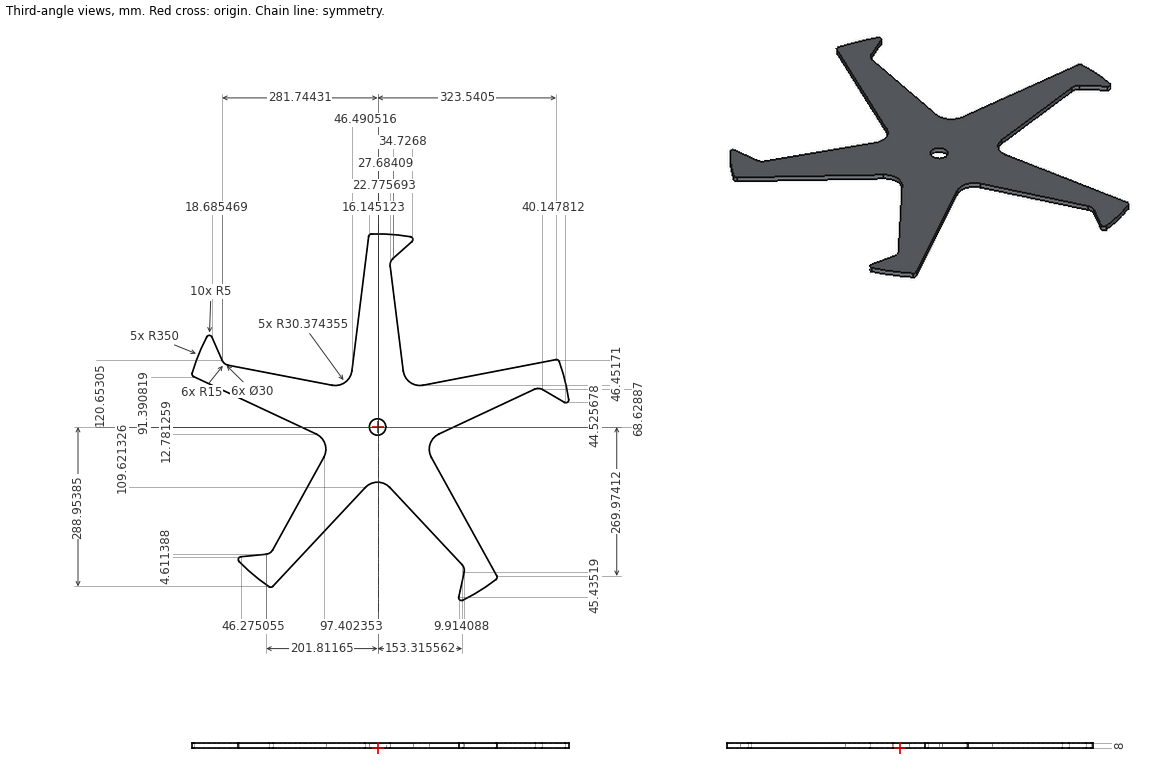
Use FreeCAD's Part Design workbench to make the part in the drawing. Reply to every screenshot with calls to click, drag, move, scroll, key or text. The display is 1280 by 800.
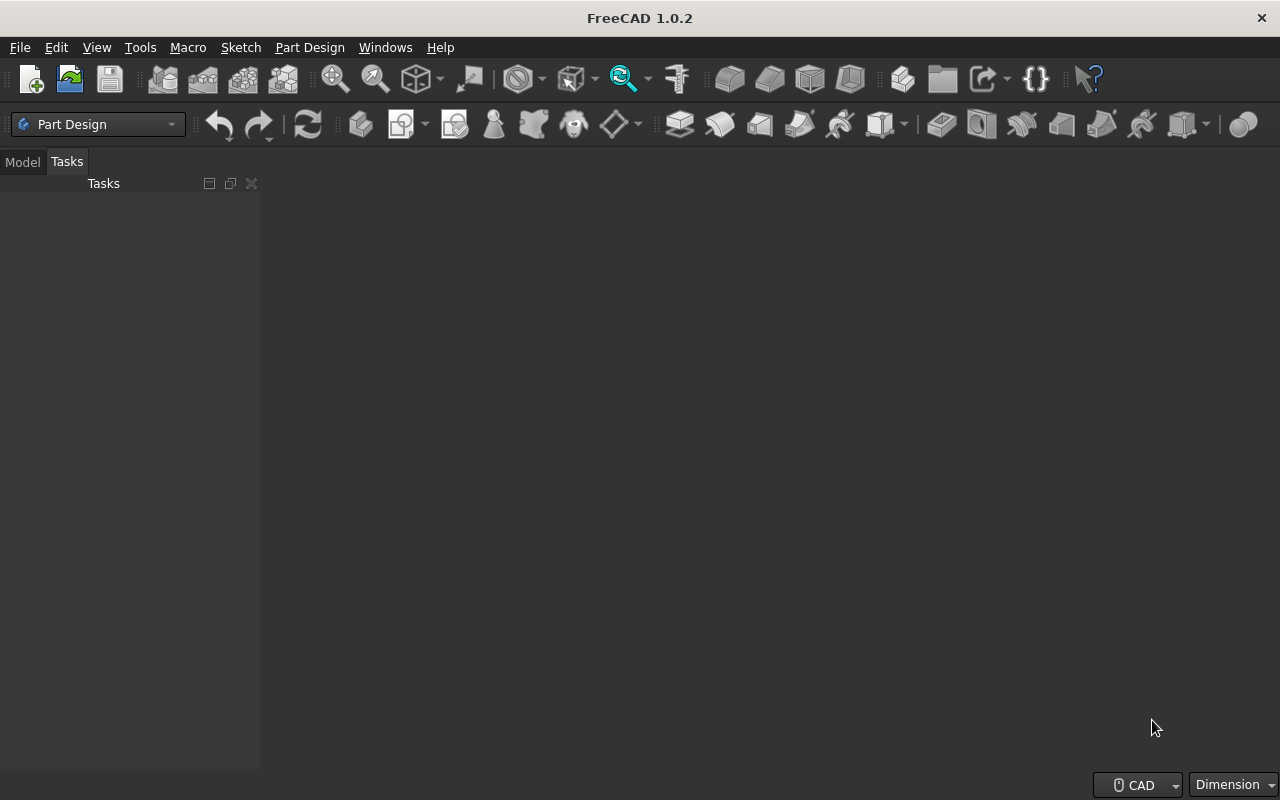
click(30, 80)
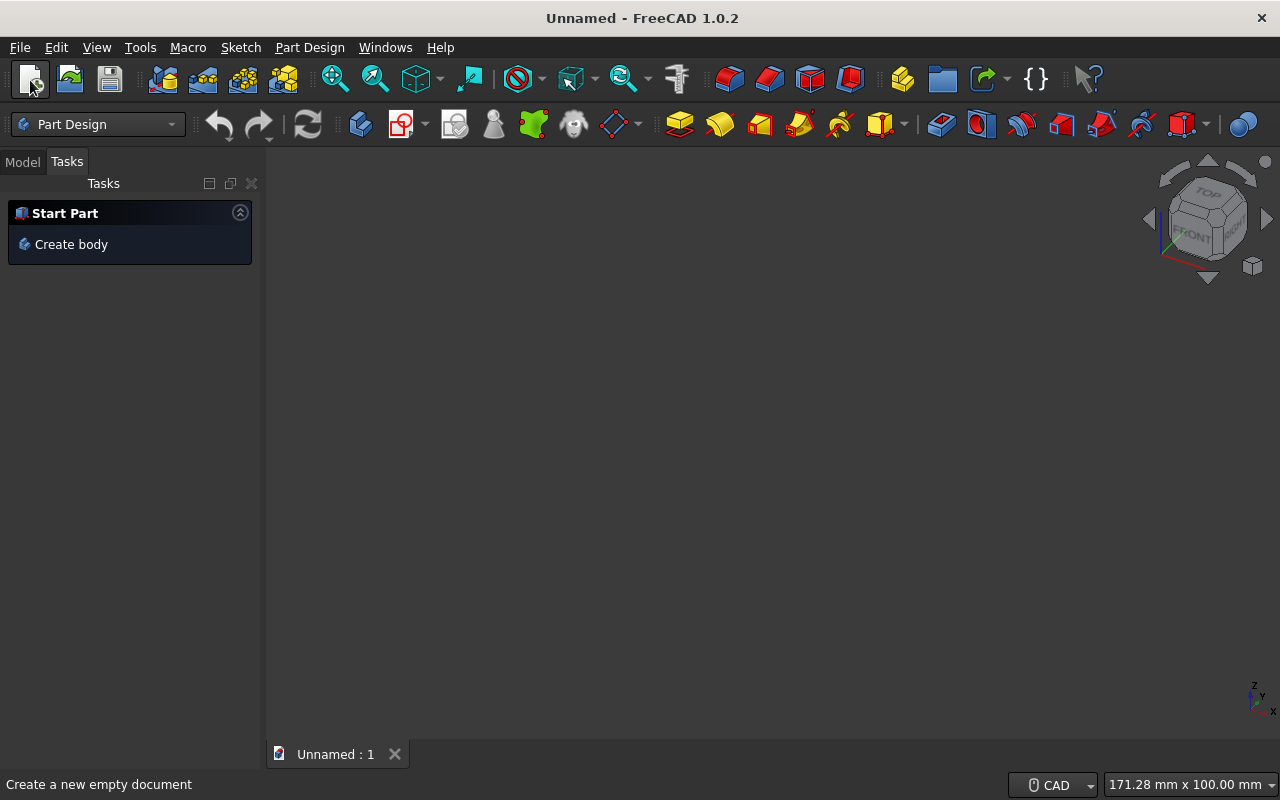
click(402, 124)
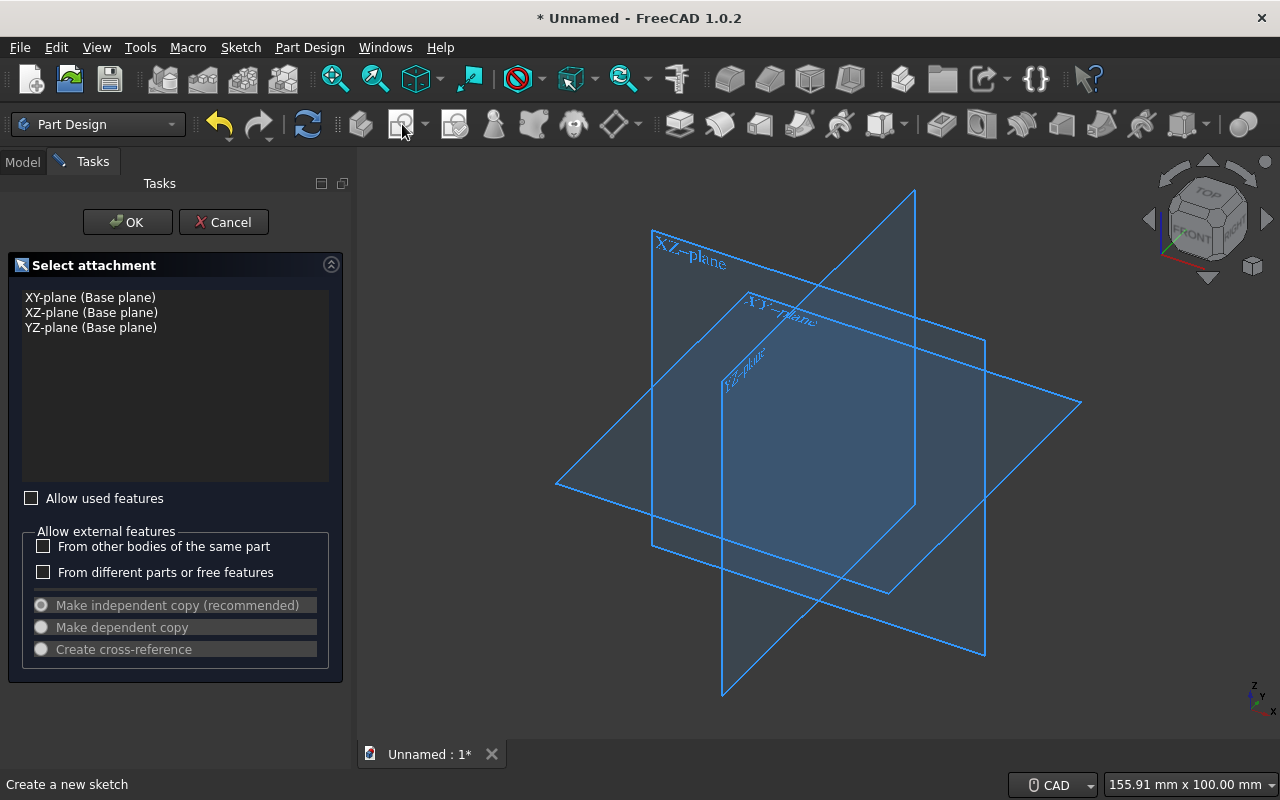
click(82, 298)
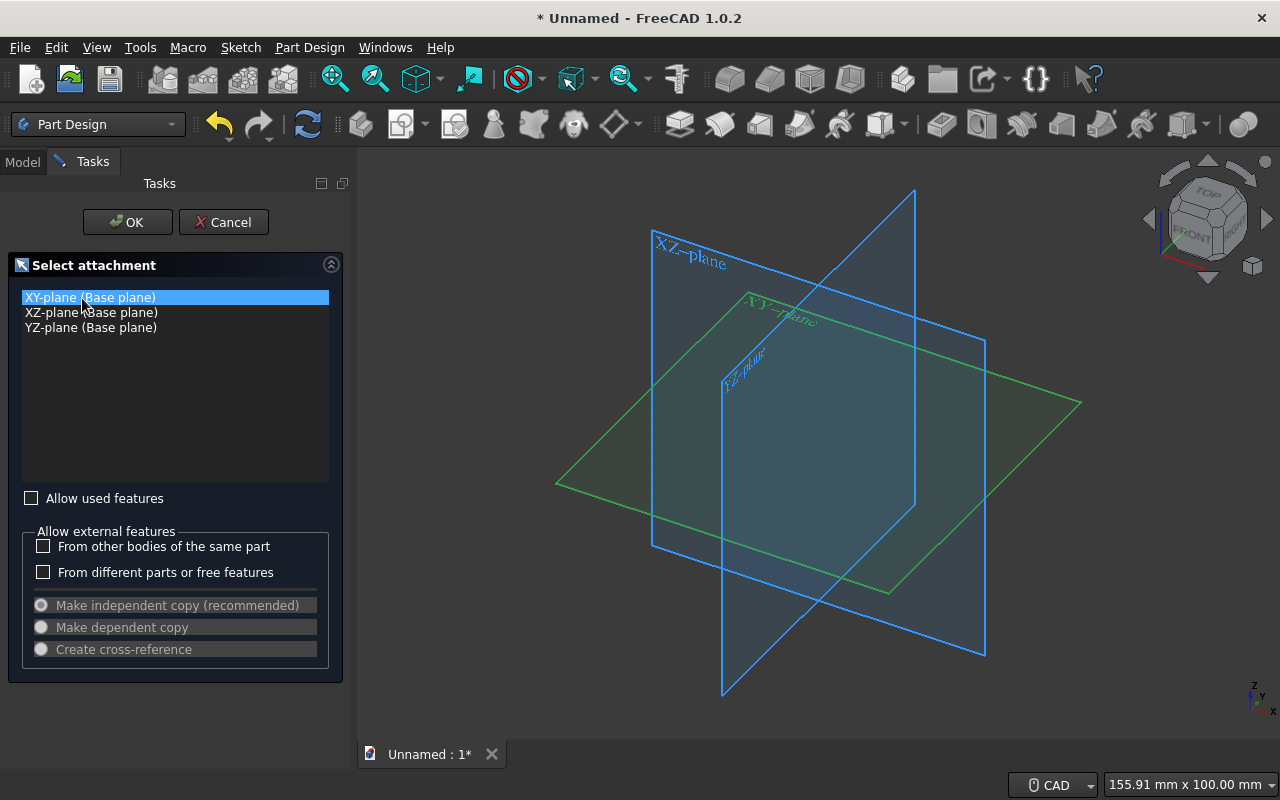
click(128, 222)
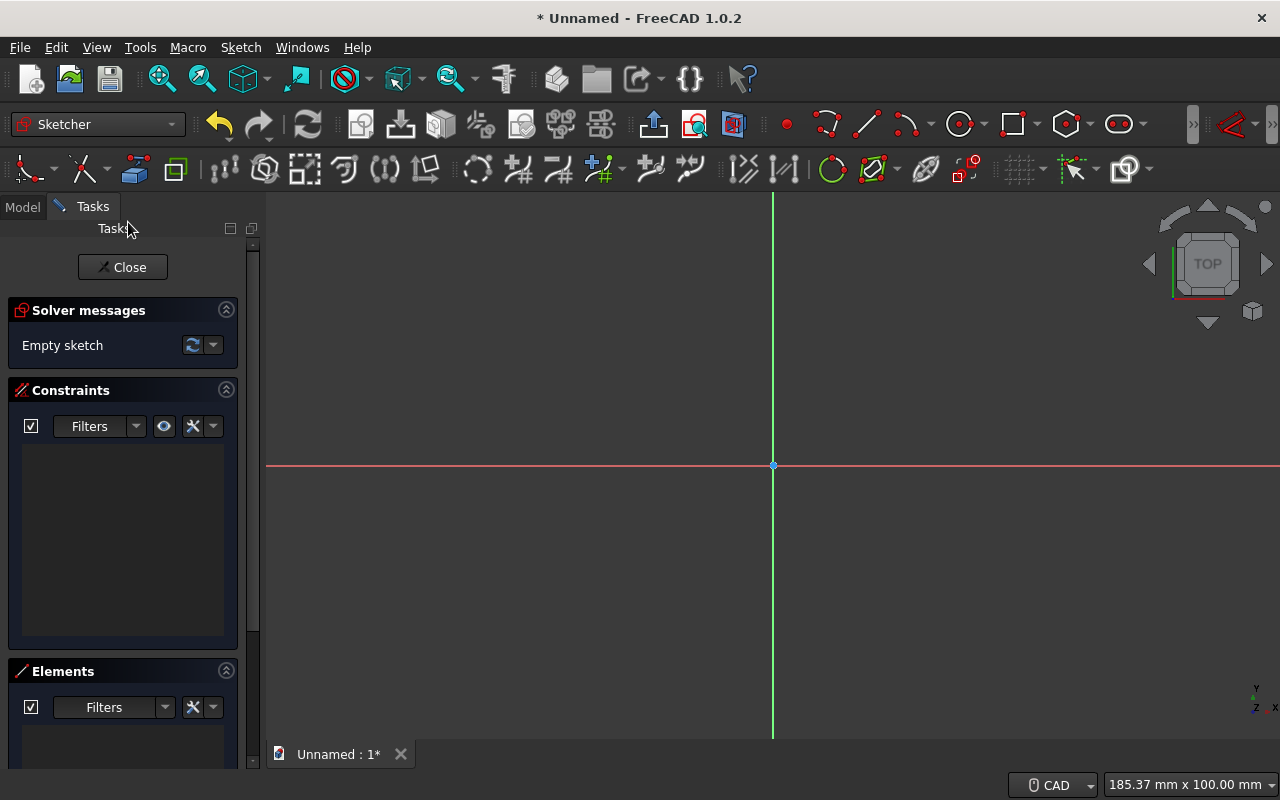
scroll(695, 475, down, 12)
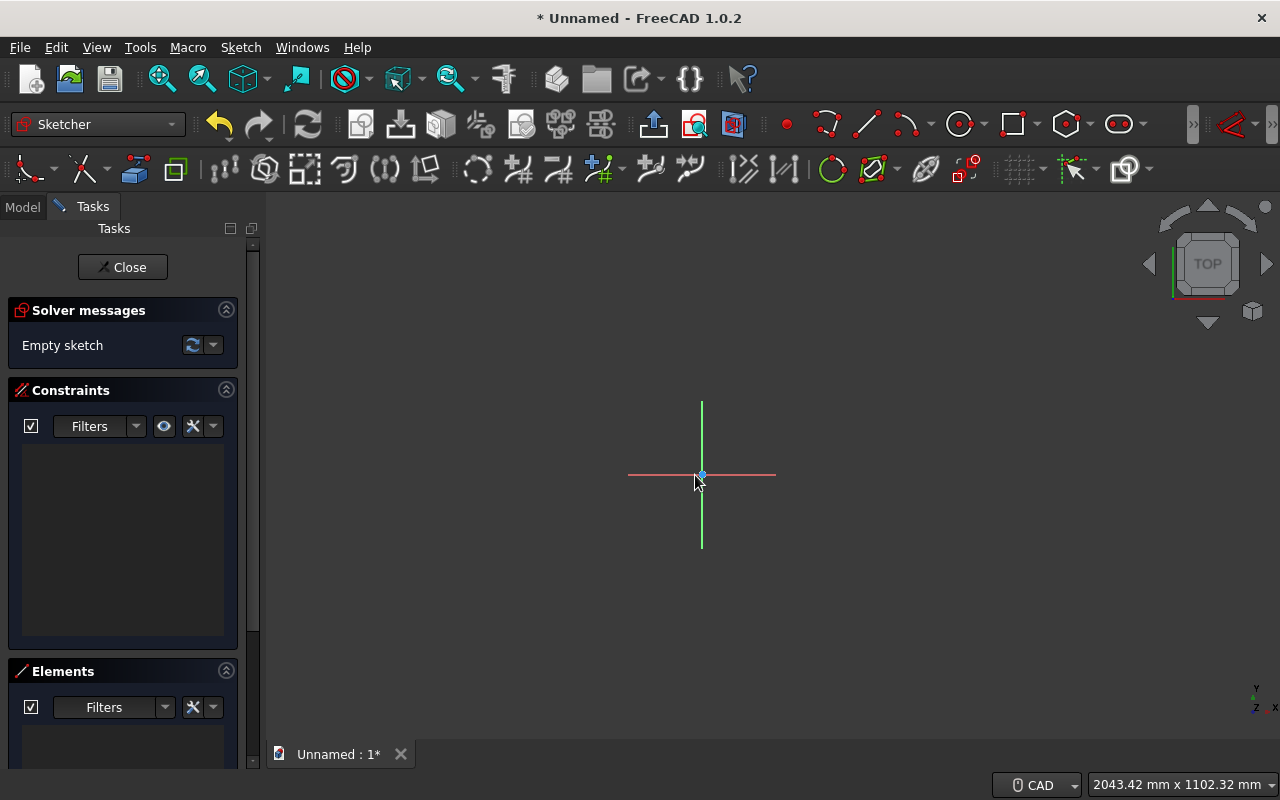
click(868, 124)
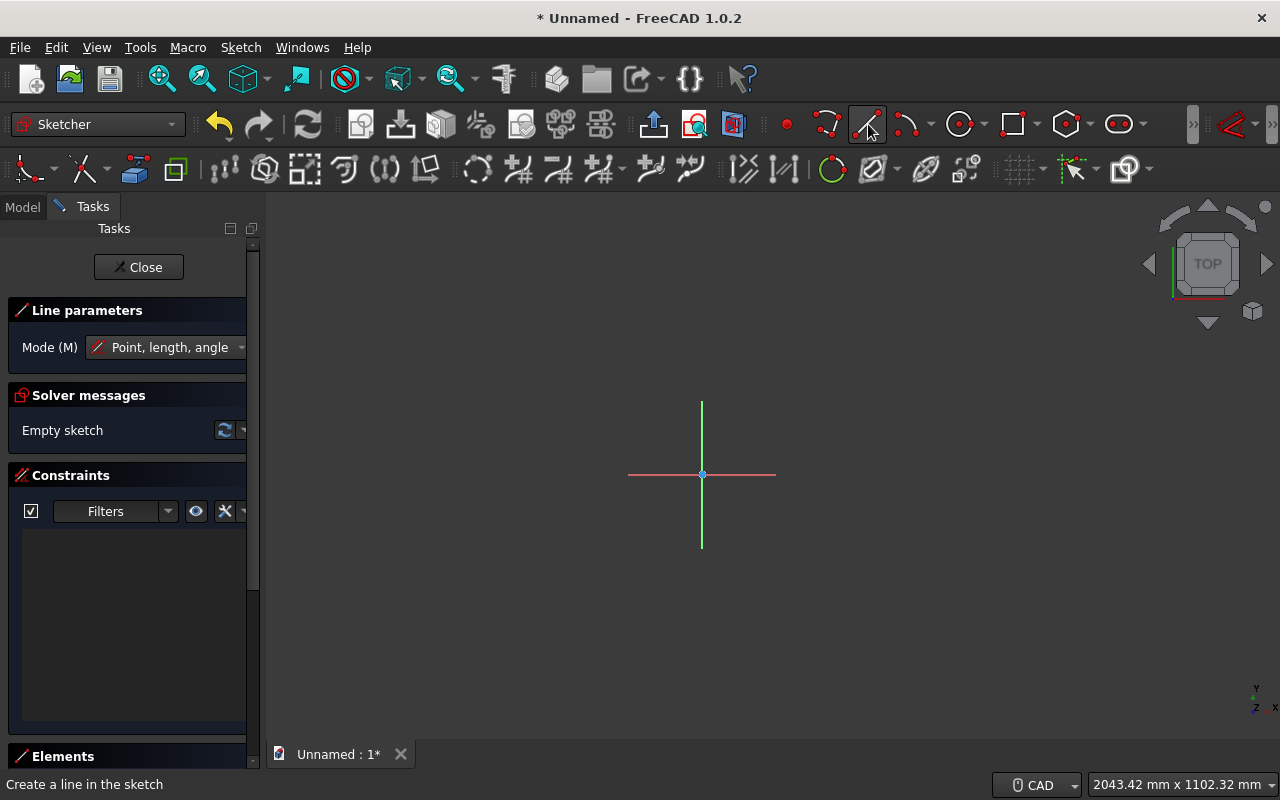
scroll(694, 303, up, 4)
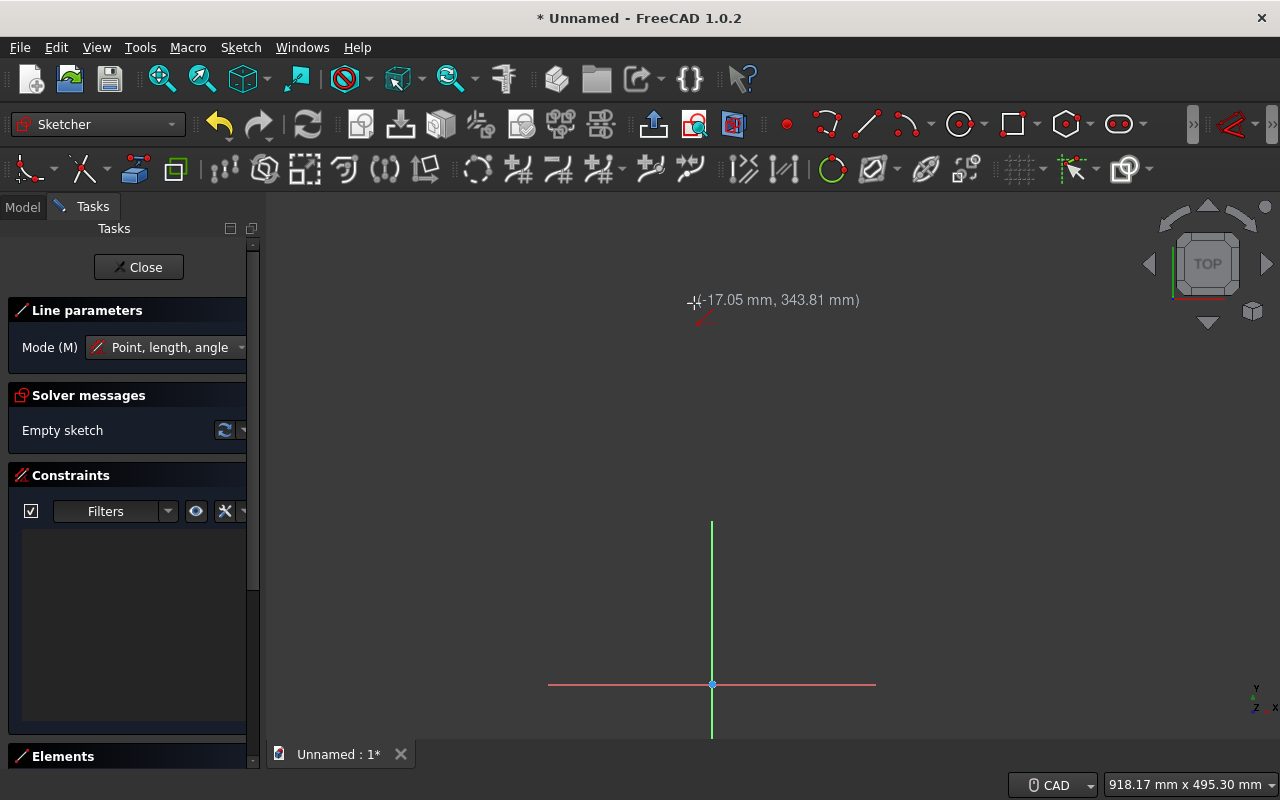
click(694, 303)
click(661, 572)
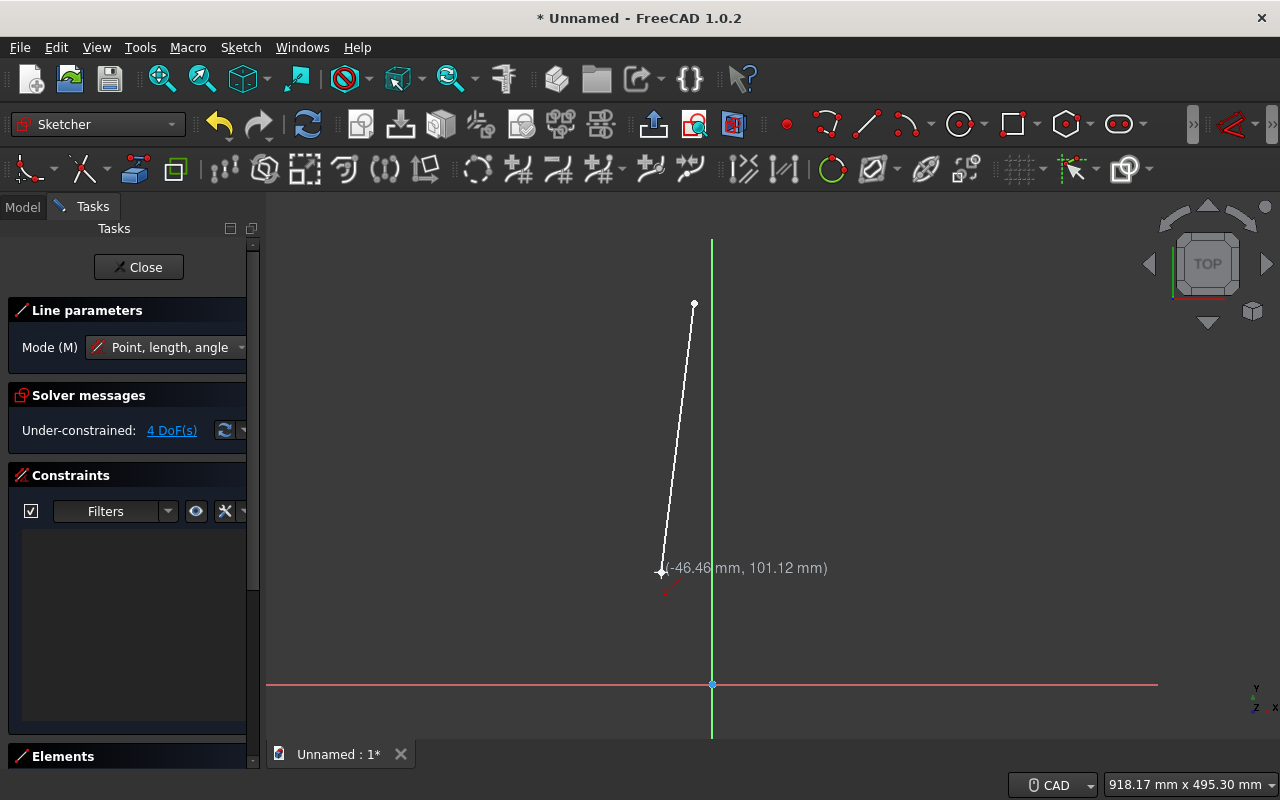
click(621, 601)
click(413, 561)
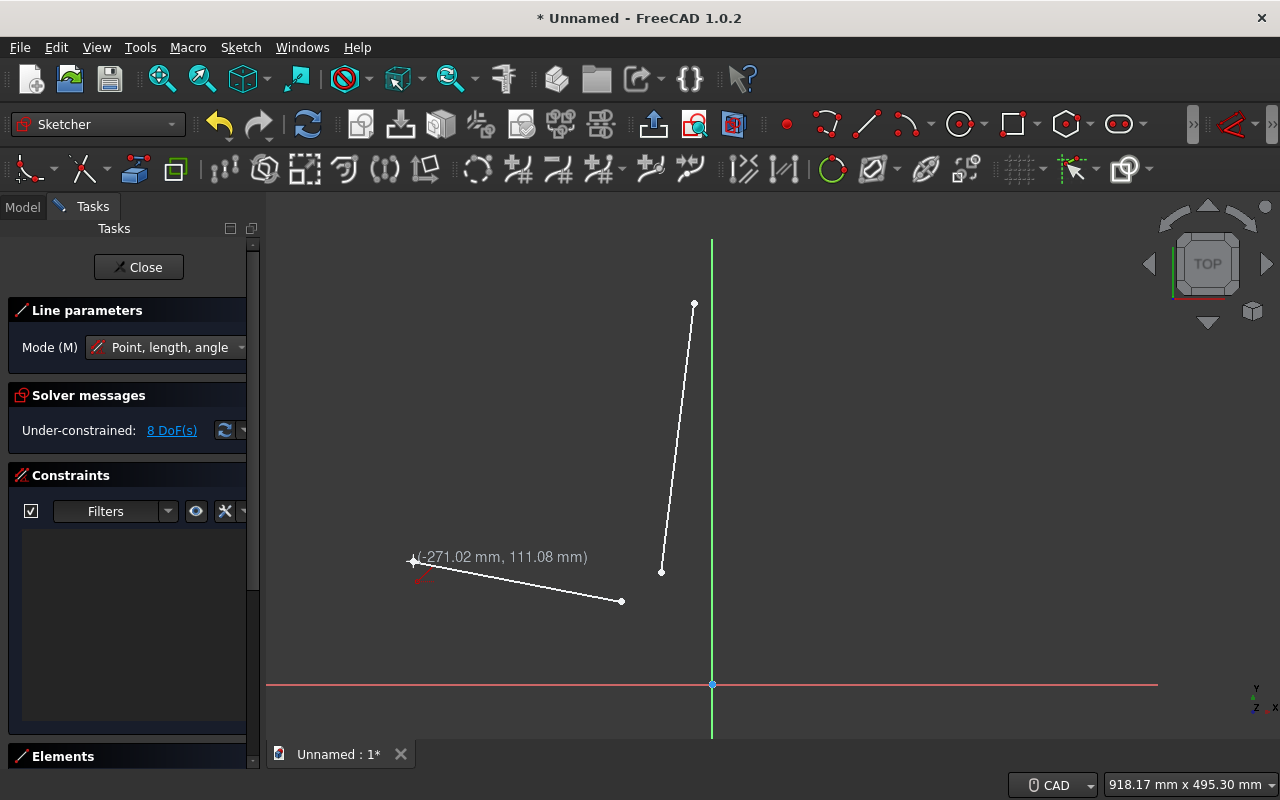
click(401, 551)
click(381, 504)